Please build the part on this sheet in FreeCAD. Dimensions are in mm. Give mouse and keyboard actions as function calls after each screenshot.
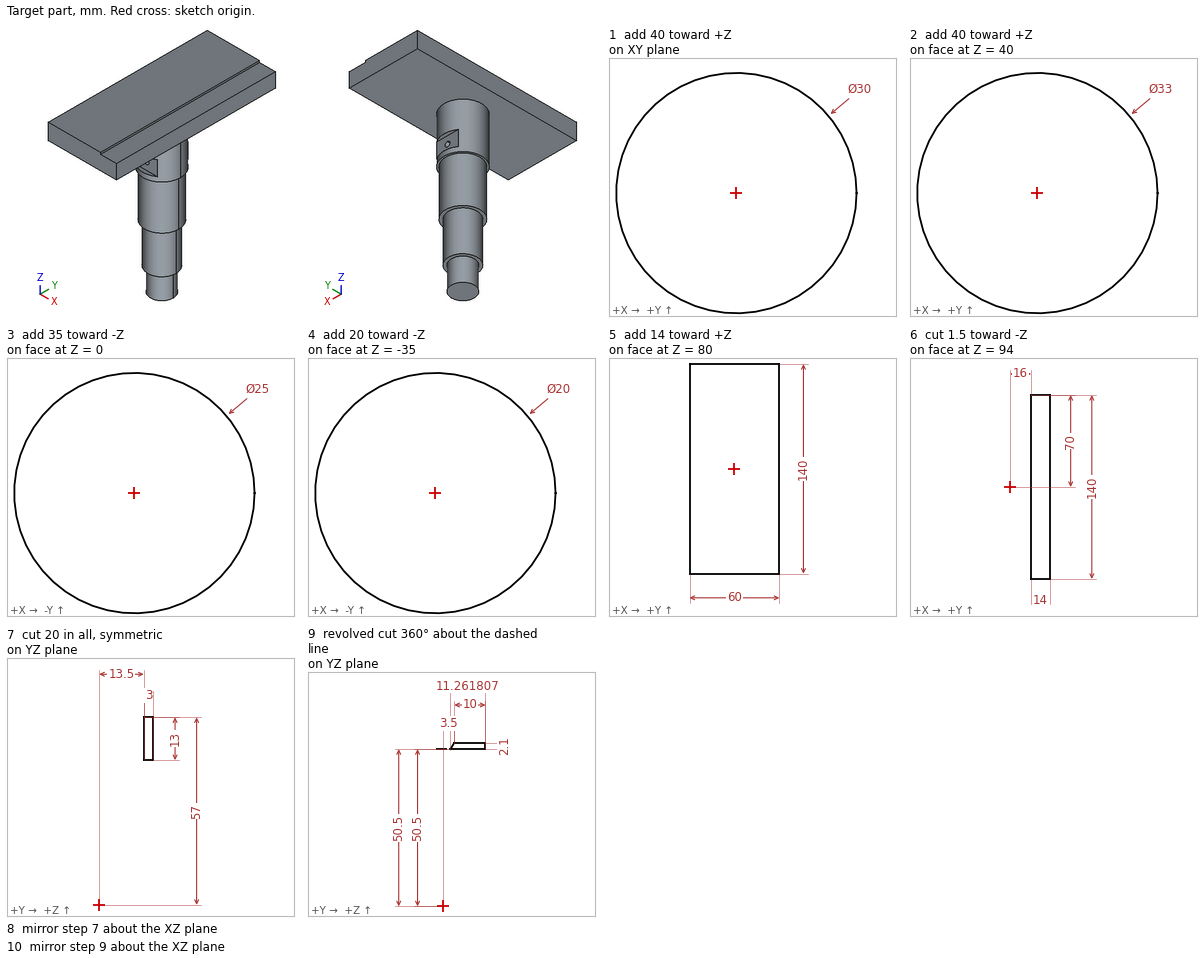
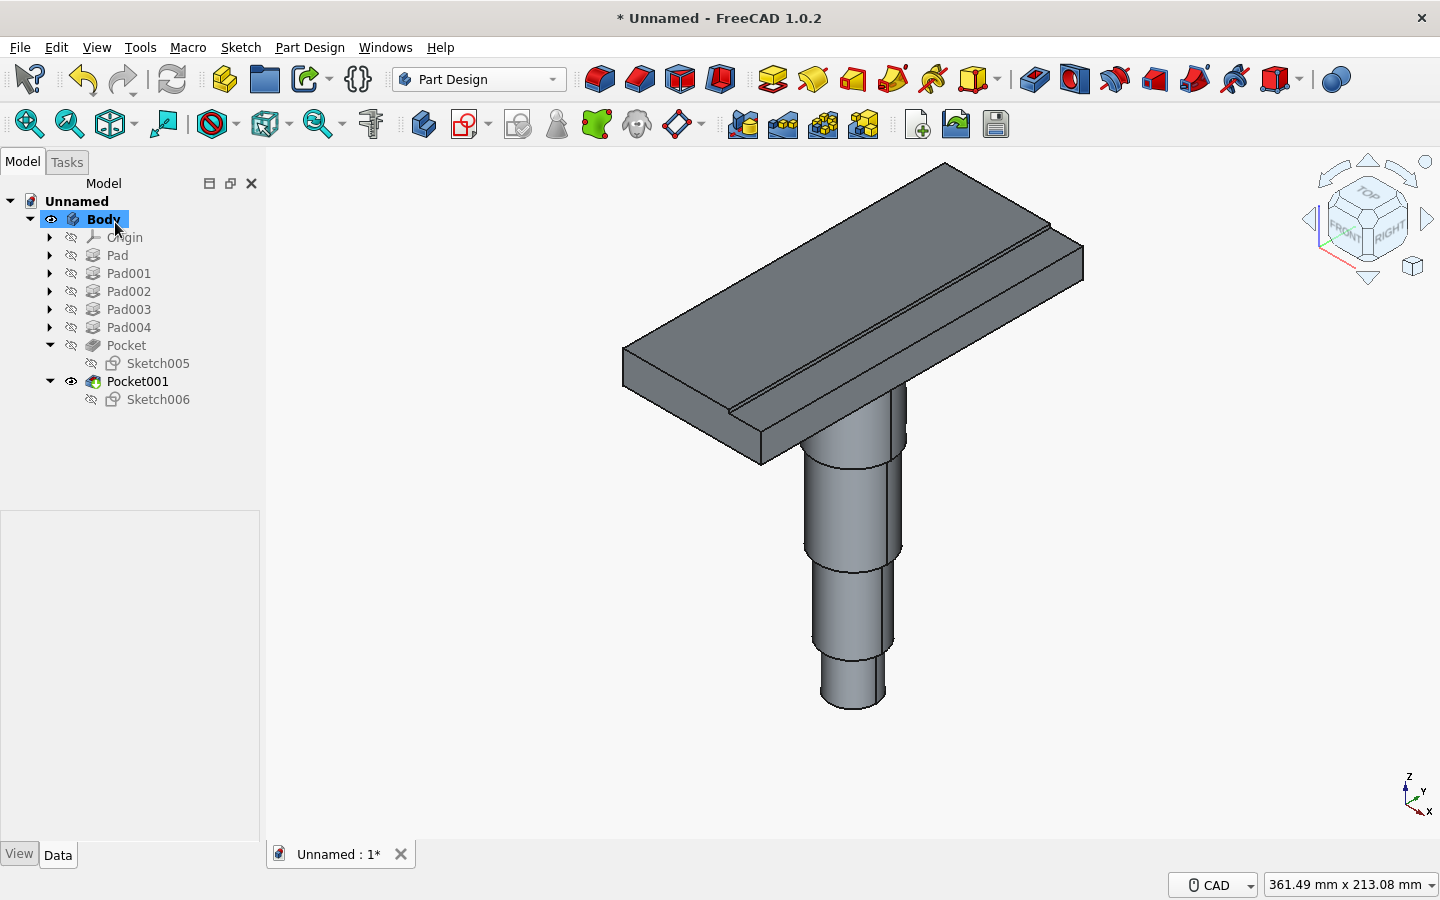
click(116, 381)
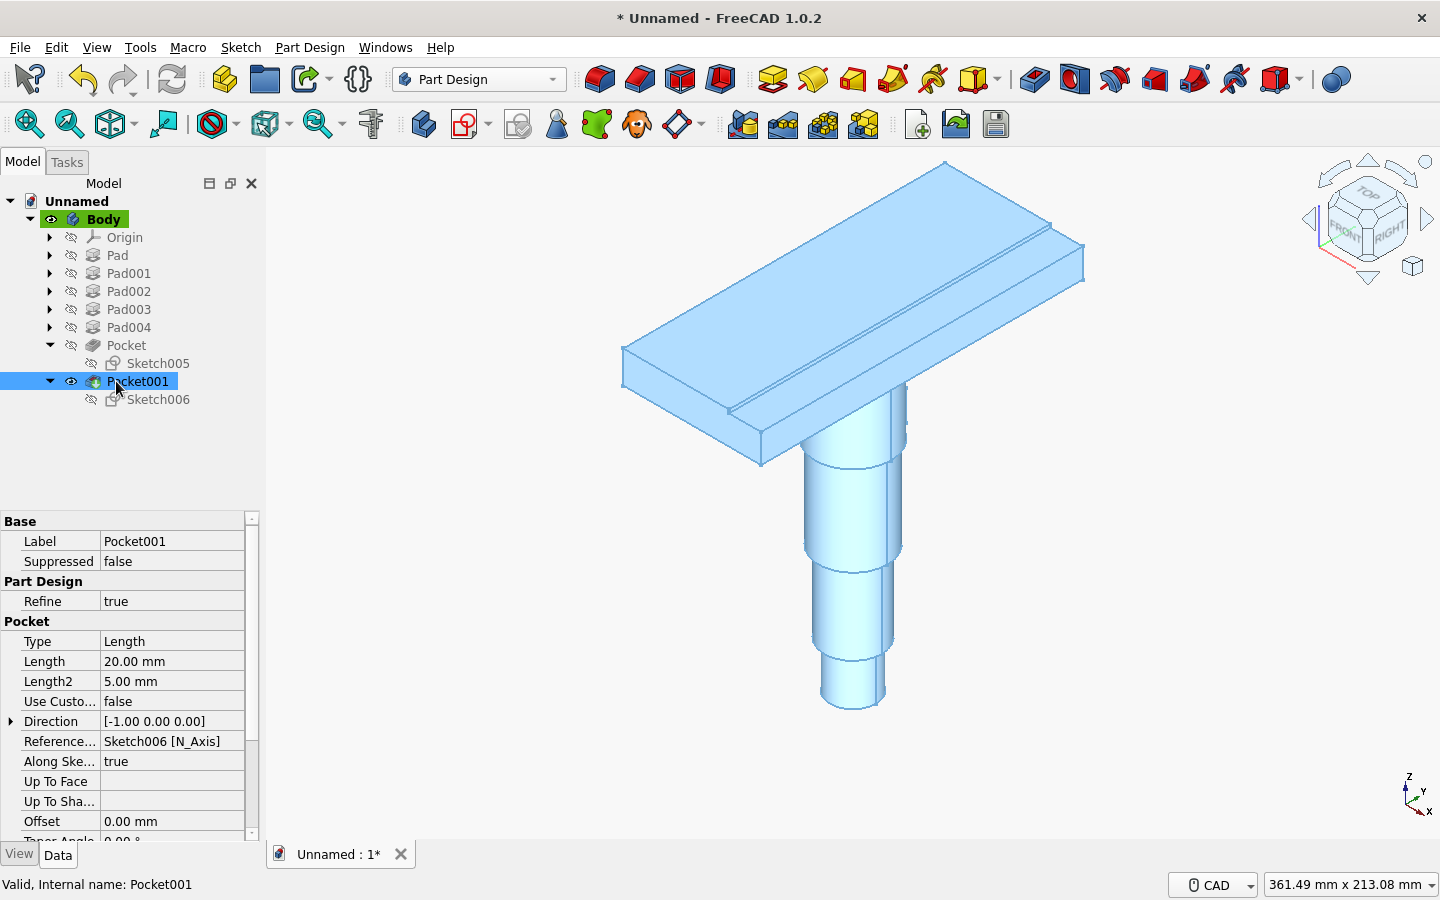
click(744, 124)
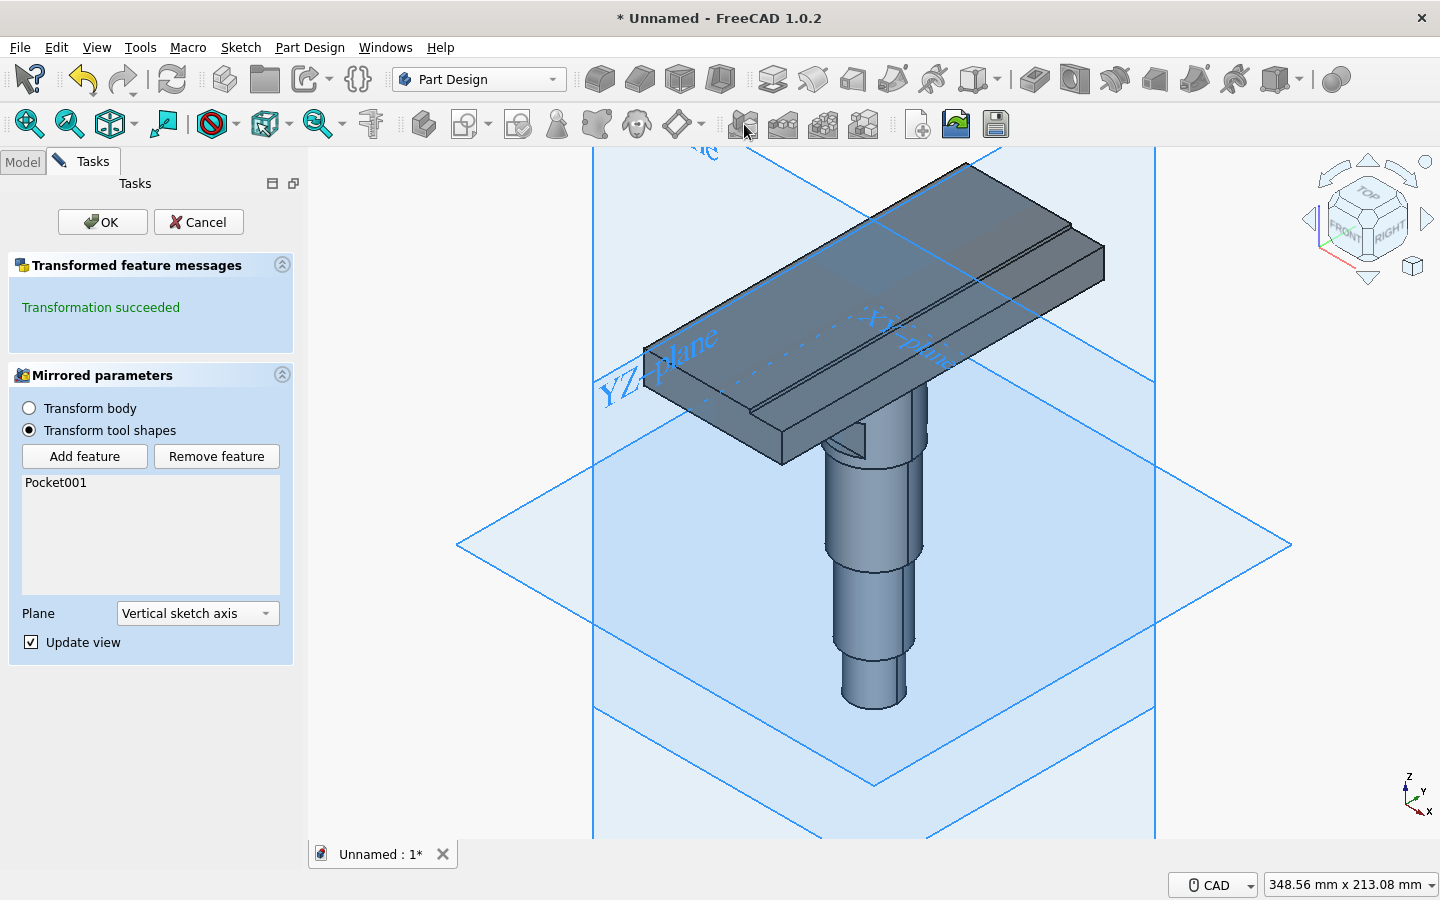
click(198, 614)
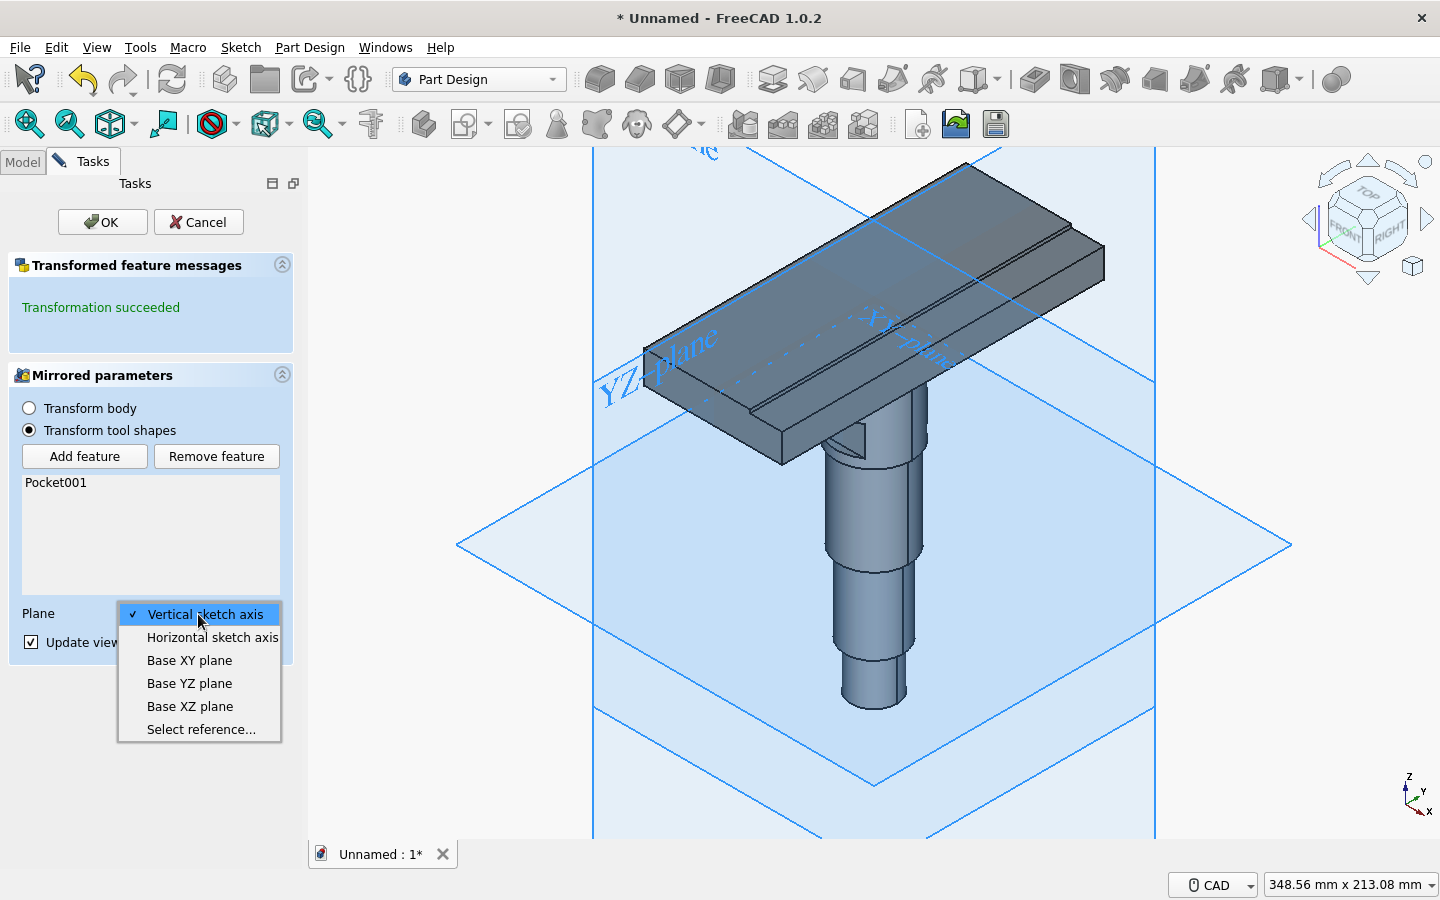
click(198, 706)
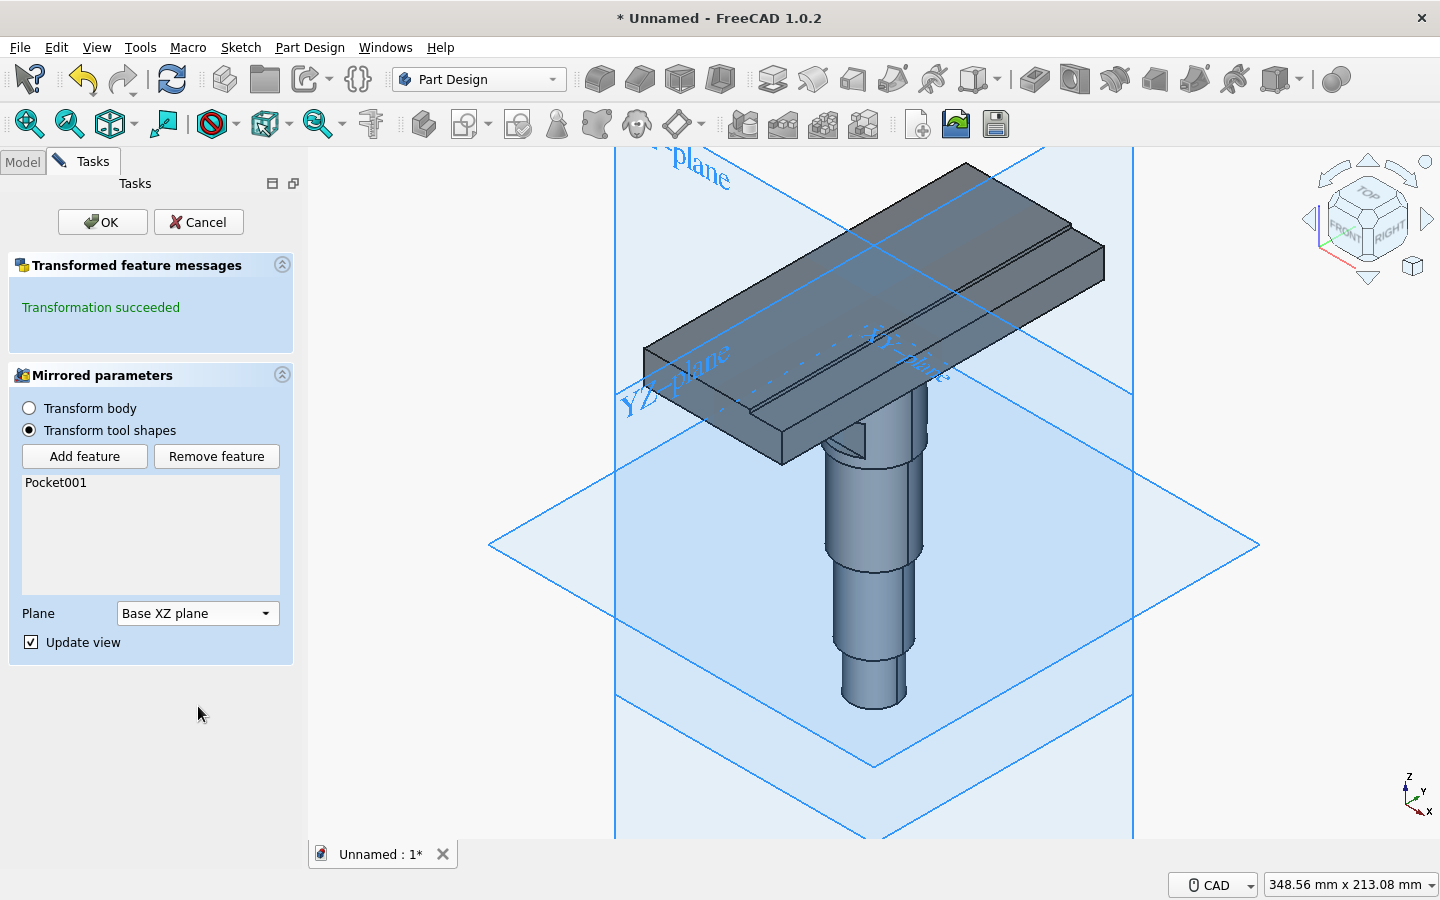
click(103, 222)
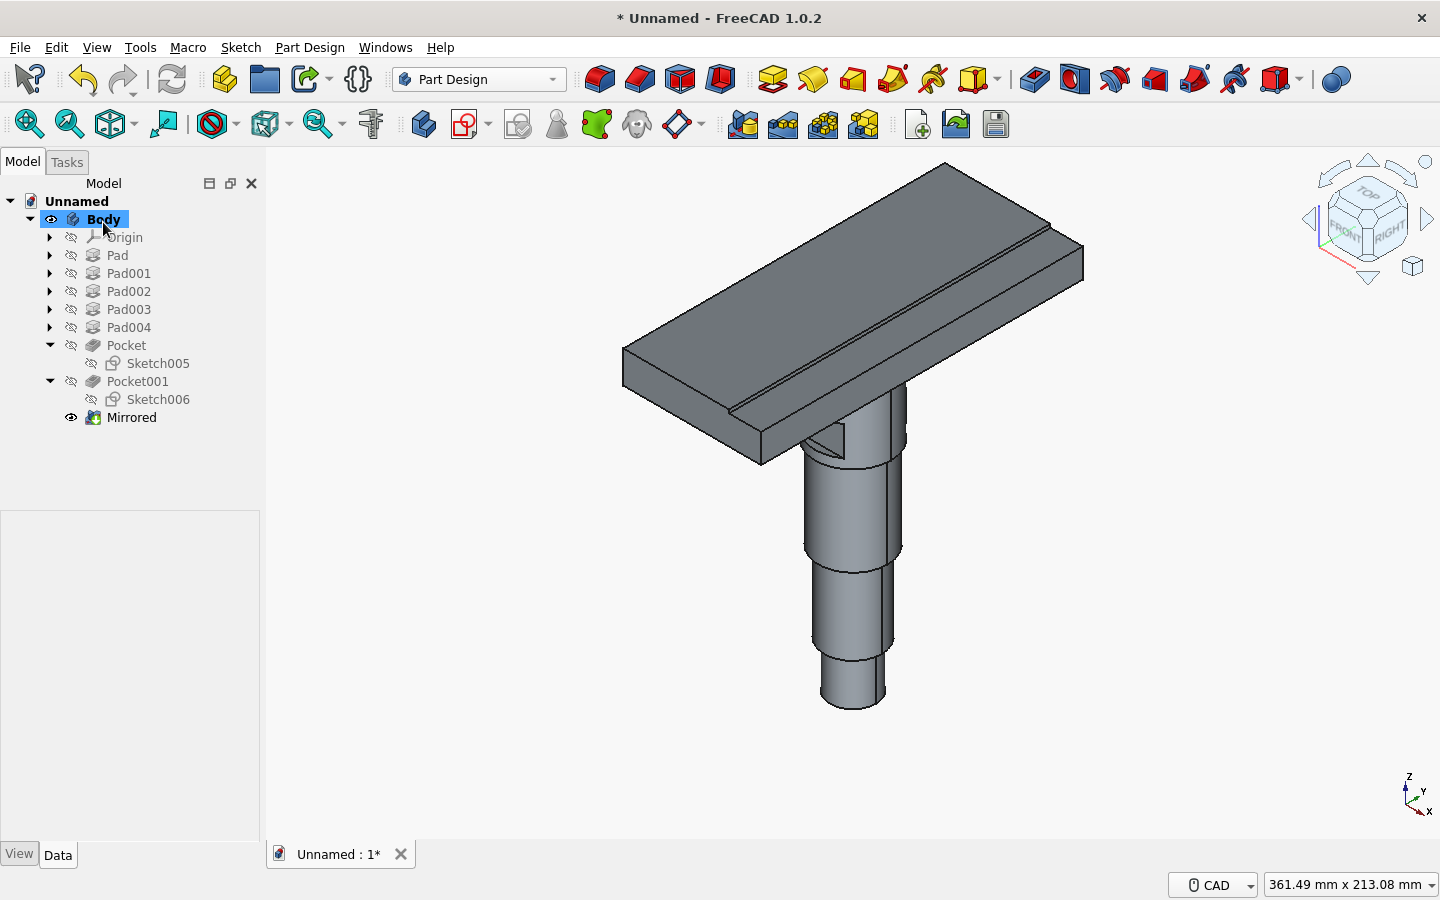
click(464, 124)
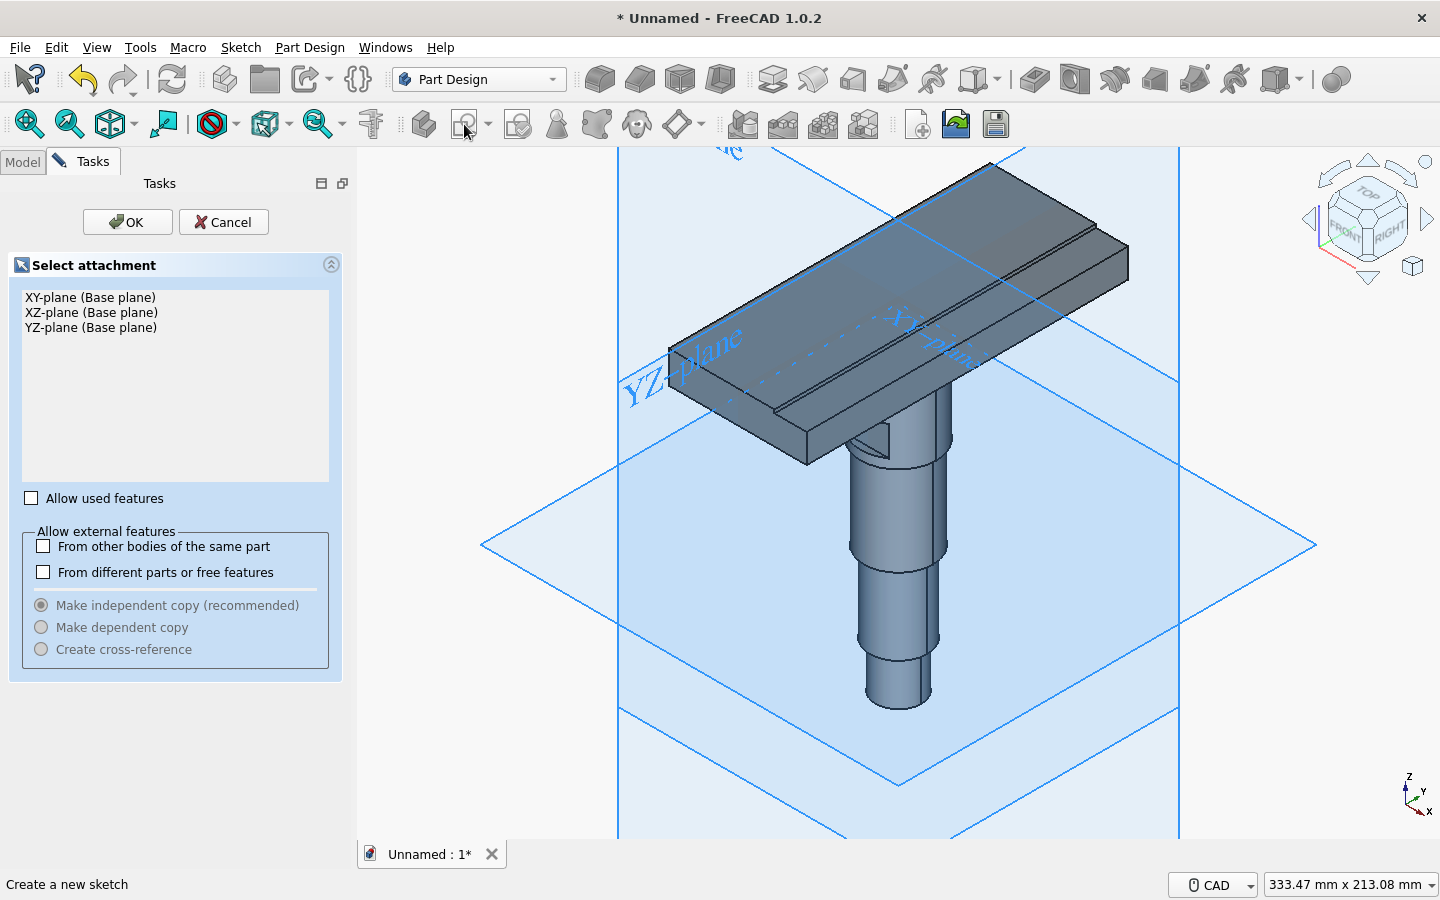
click(82, 328)